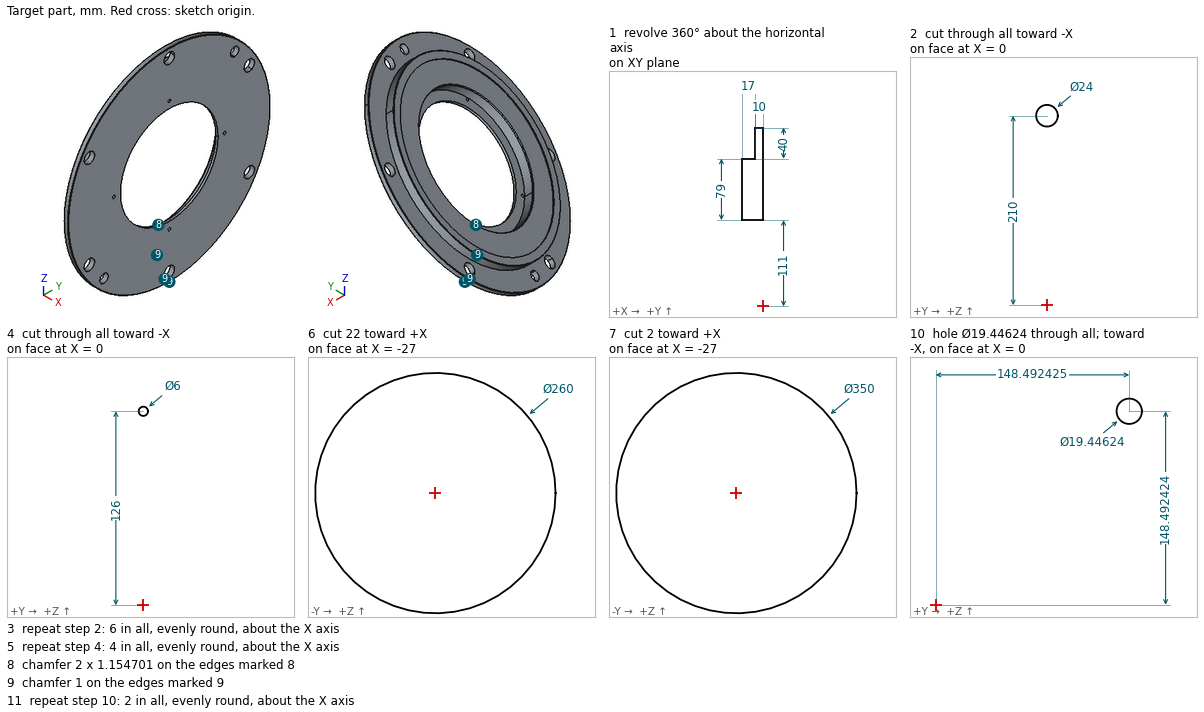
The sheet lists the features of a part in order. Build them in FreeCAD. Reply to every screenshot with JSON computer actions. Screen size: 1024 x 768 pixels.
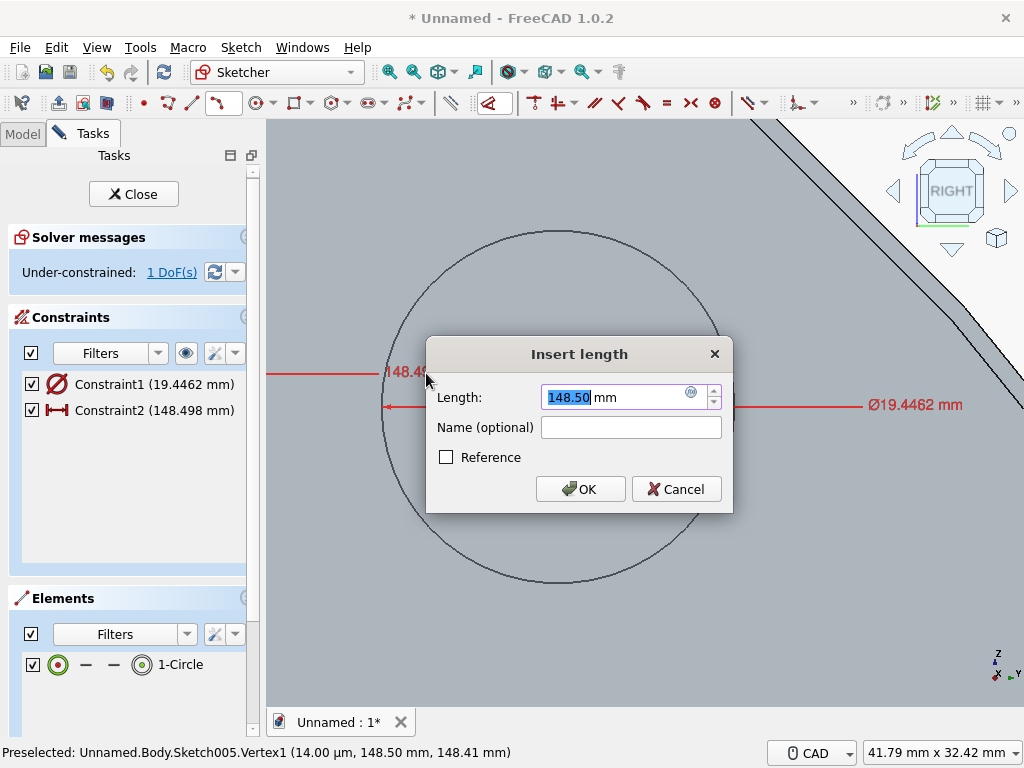
{"action": "type", "text": "148.492425"}
{"action": "key", "text": "Return"}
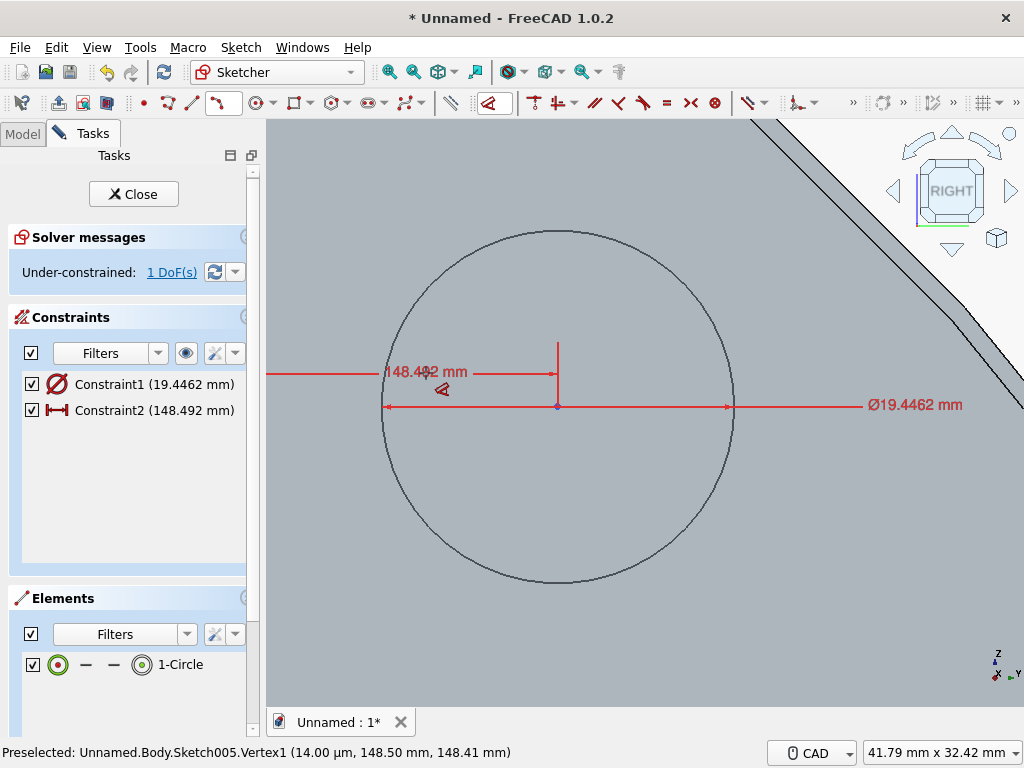
{"action": "left_click", "coordinate": [558, 407]}
{"action": "left_click", "coordinate": [592, 543]}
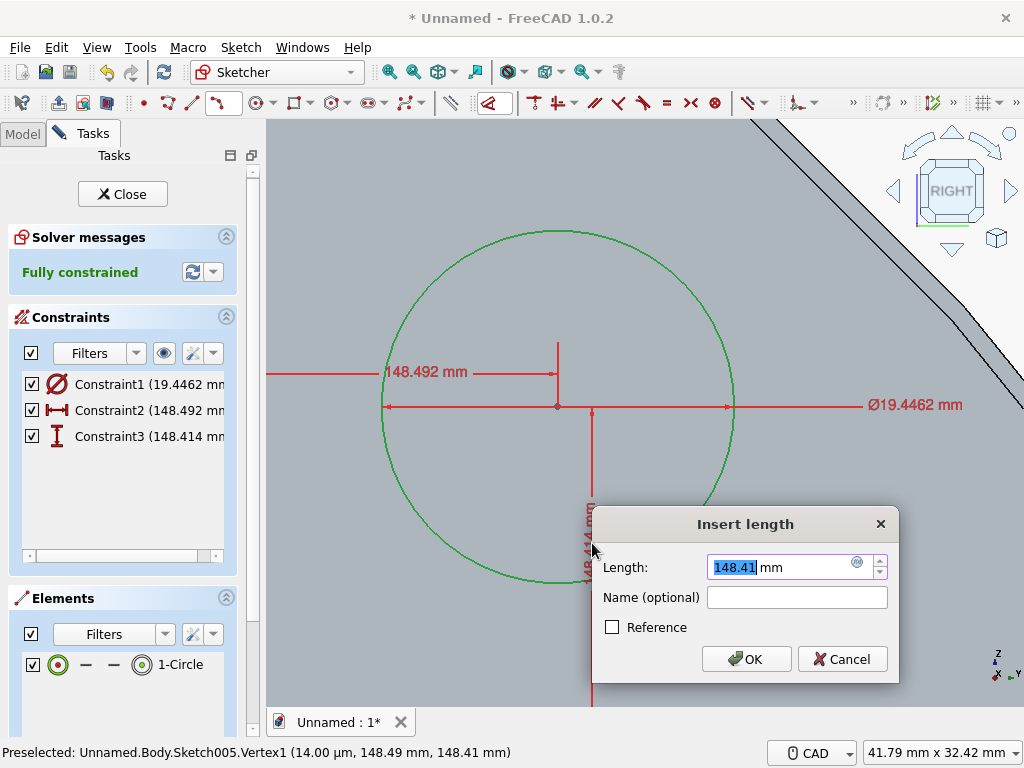
{"action": "type", "text": "148.492424"}
{"action": "key", "text": "Return"}
{"action": "key", "text": "Escape"}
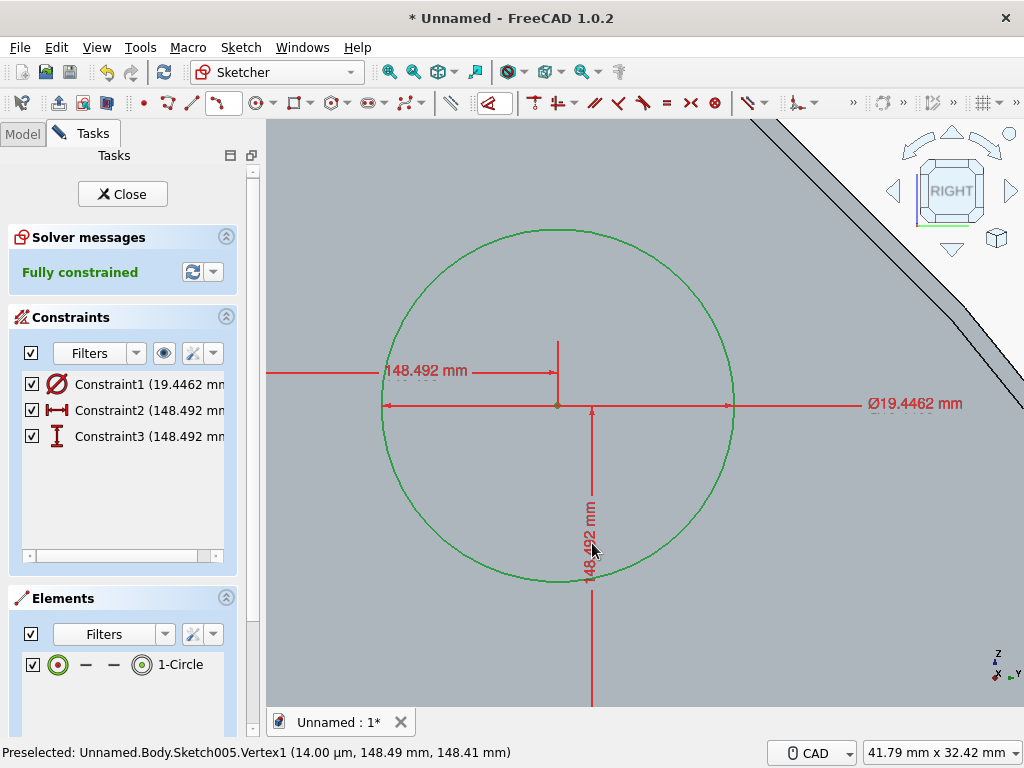
{"action": "left_click", "coordinate": [123, 194]}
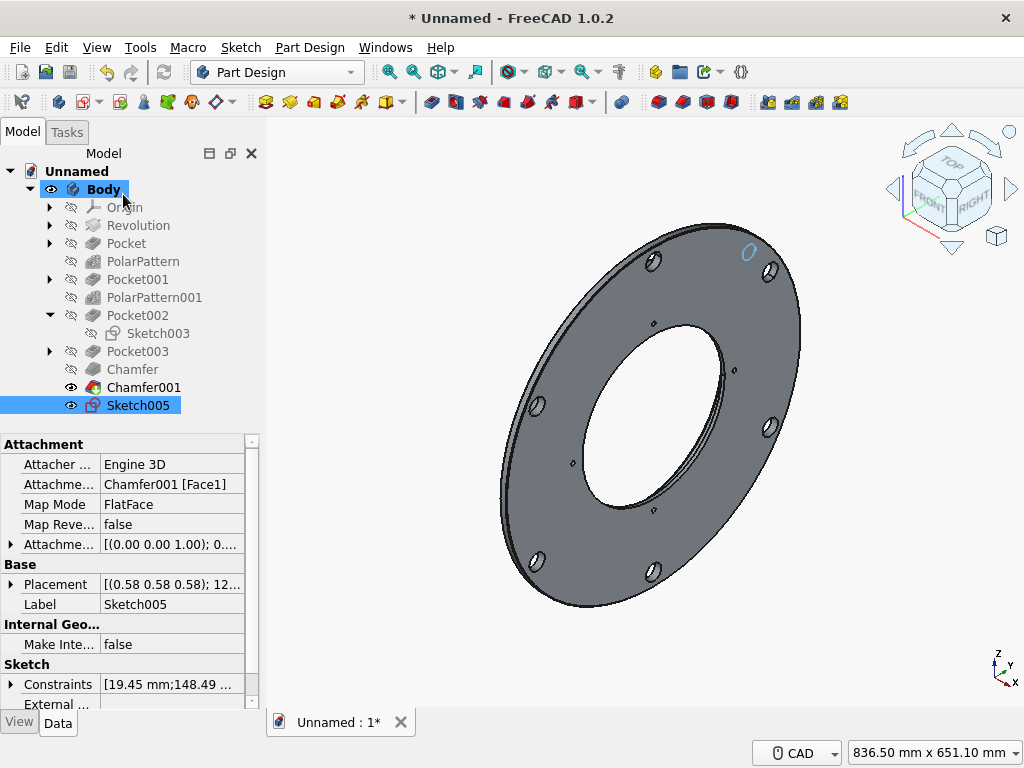
{"action": "left_click", "coordinate": [456, 102]}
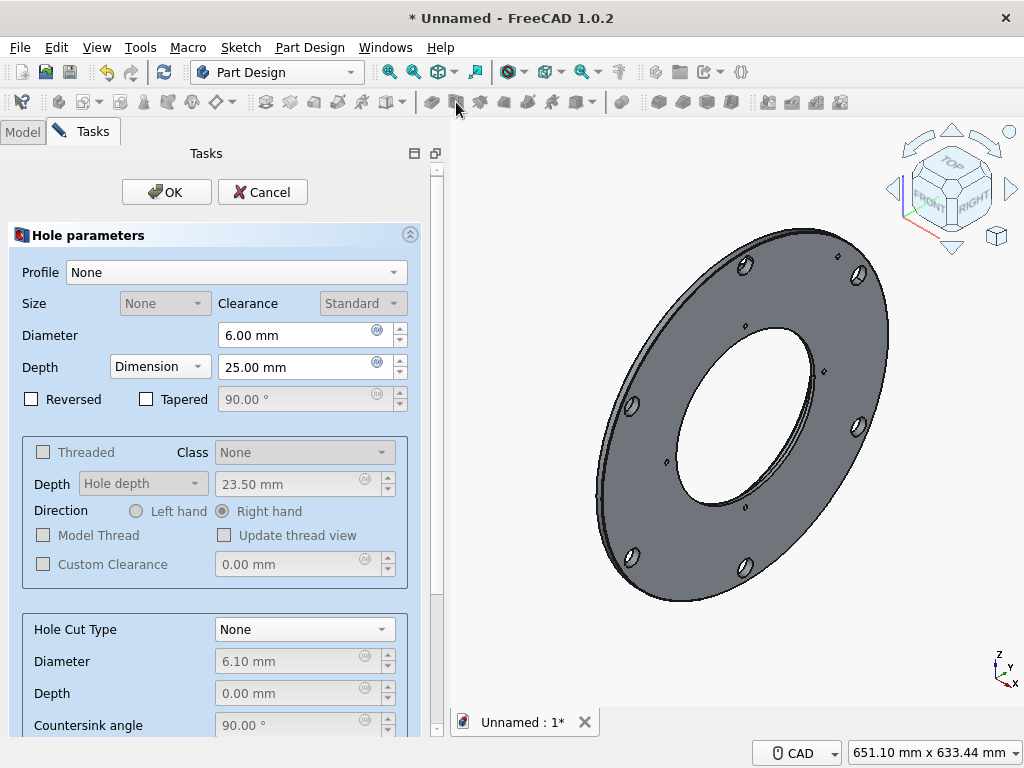
{"action": "triple_click", "coordinate": [305, 335]}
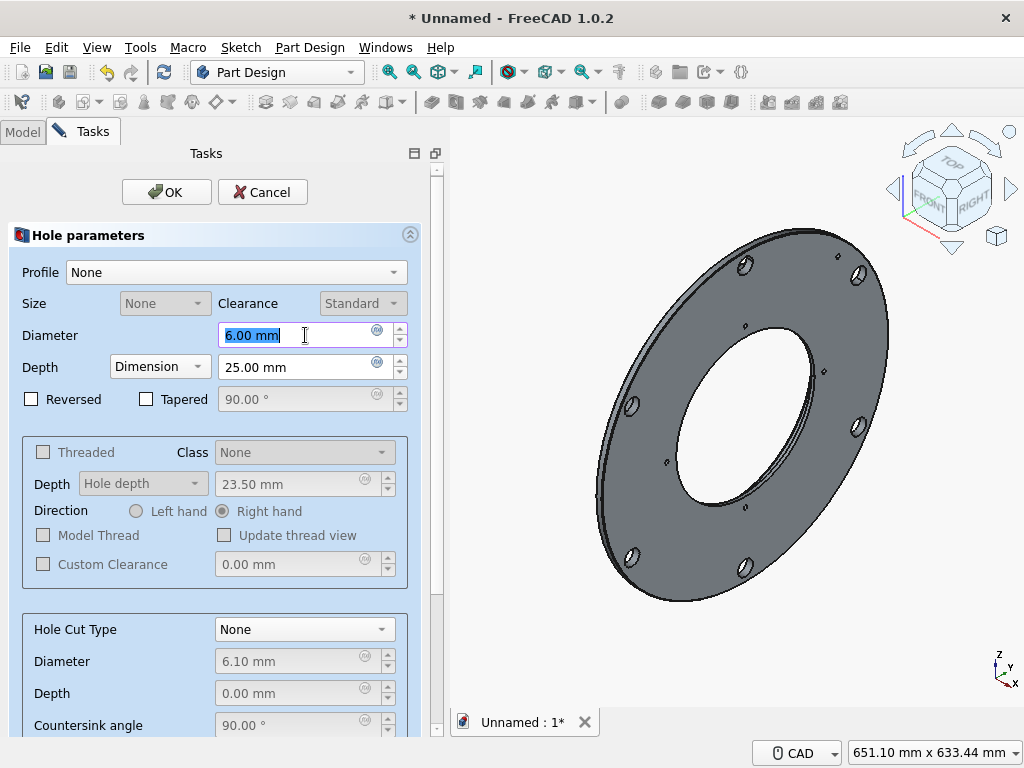
{"action": "type", "text": "19.44624"}
{"action": "key", "text": "Tab"}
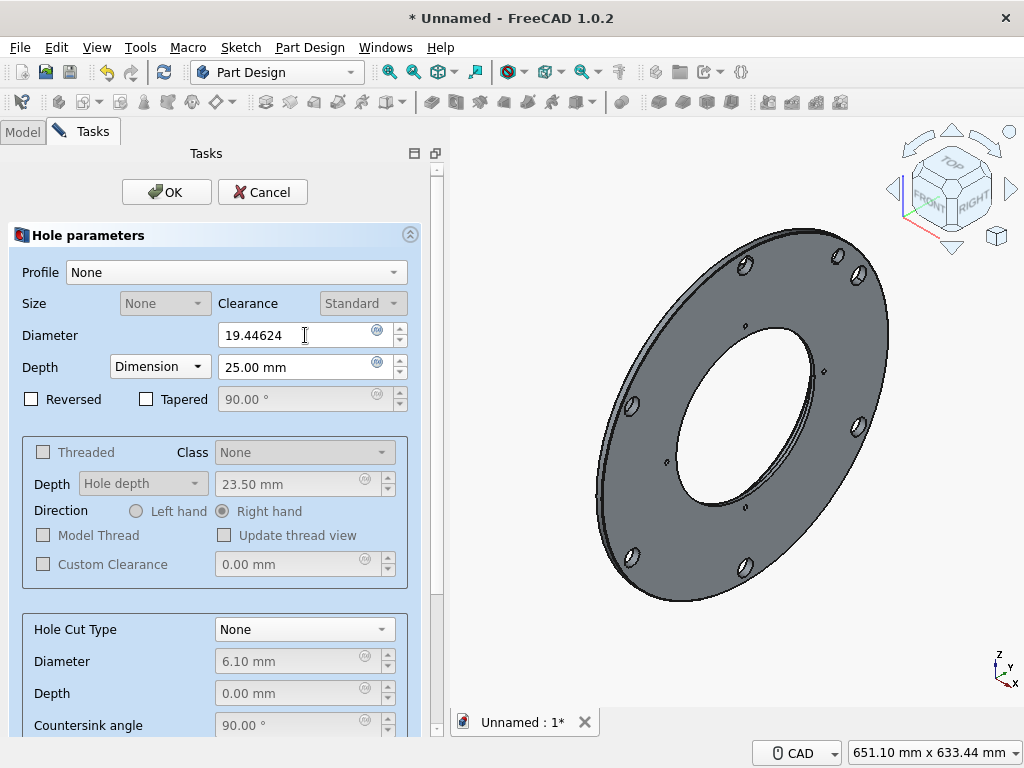
{"action": "left_click", "coordinate": [161, 366]}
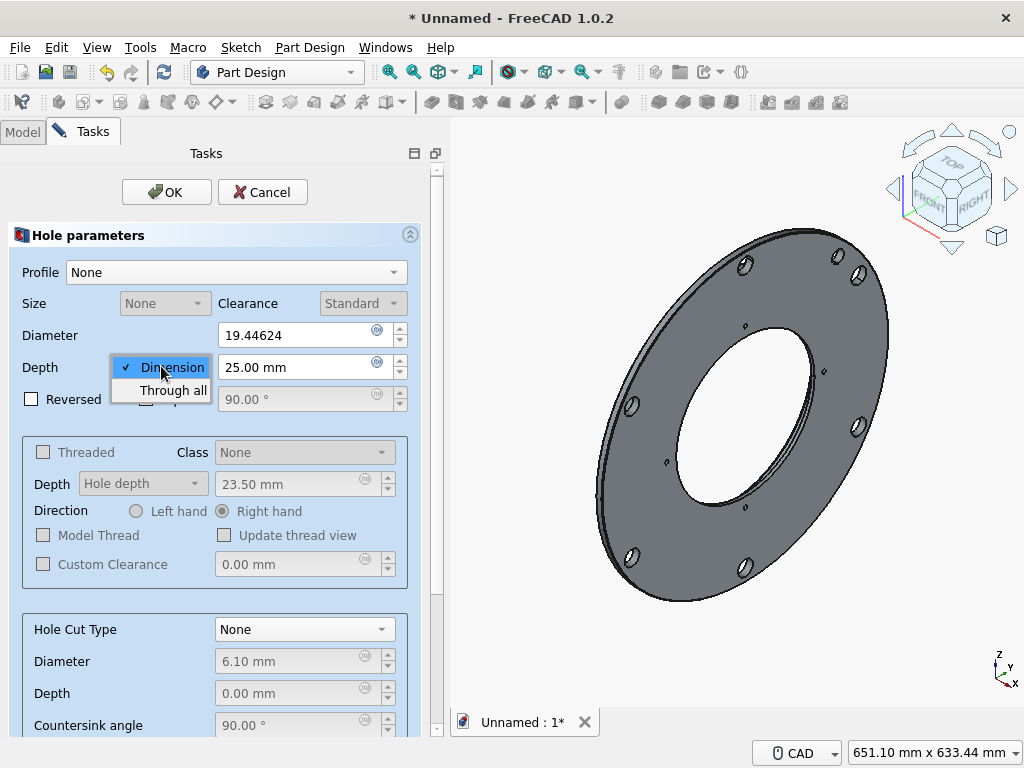
{"action": "left_click", "coordinate": [160, 390]}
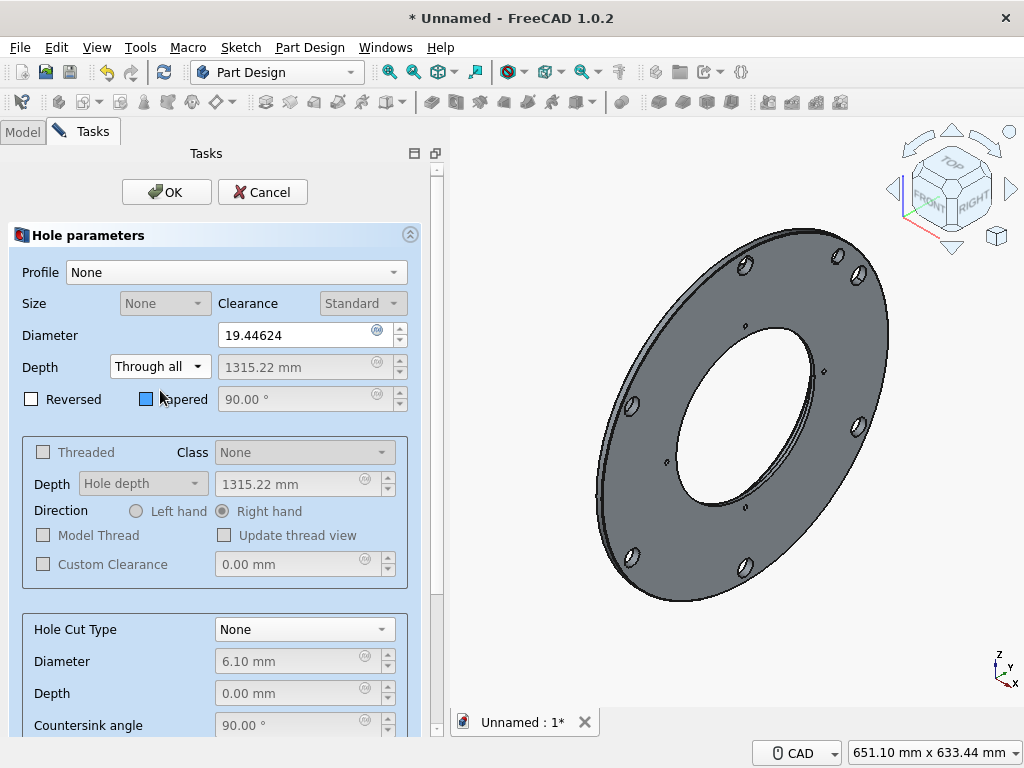
{"action": "left_click", "coordinate": [167, 192]}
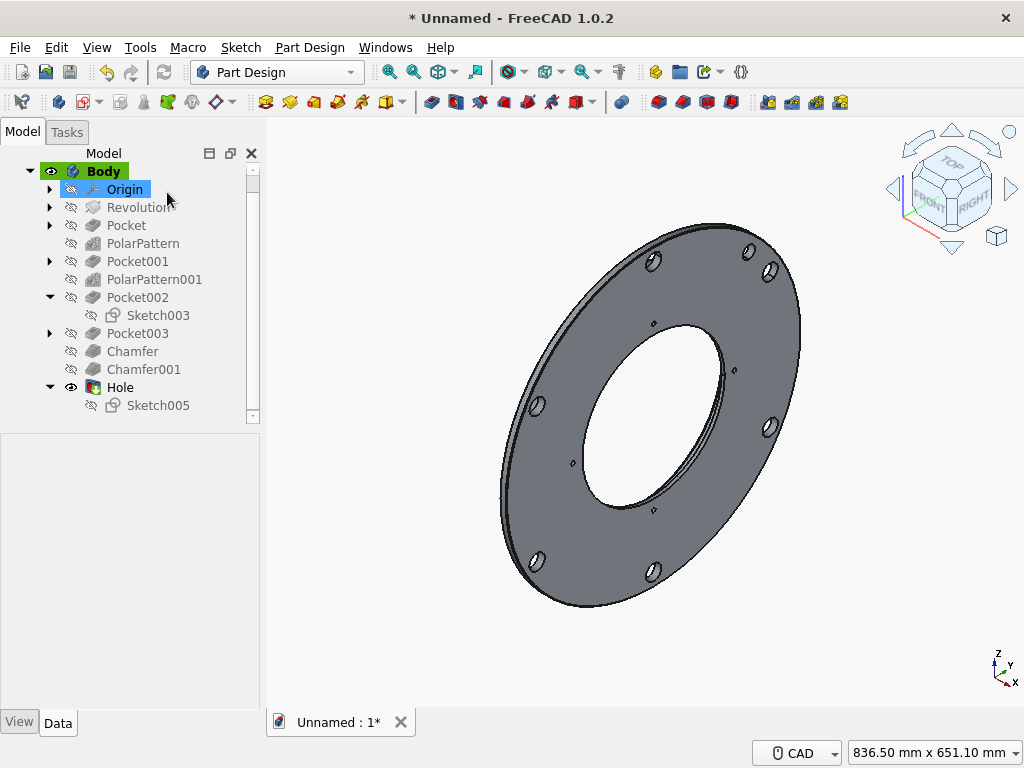
{"action": "left_click", "coordinate": [116, 387]}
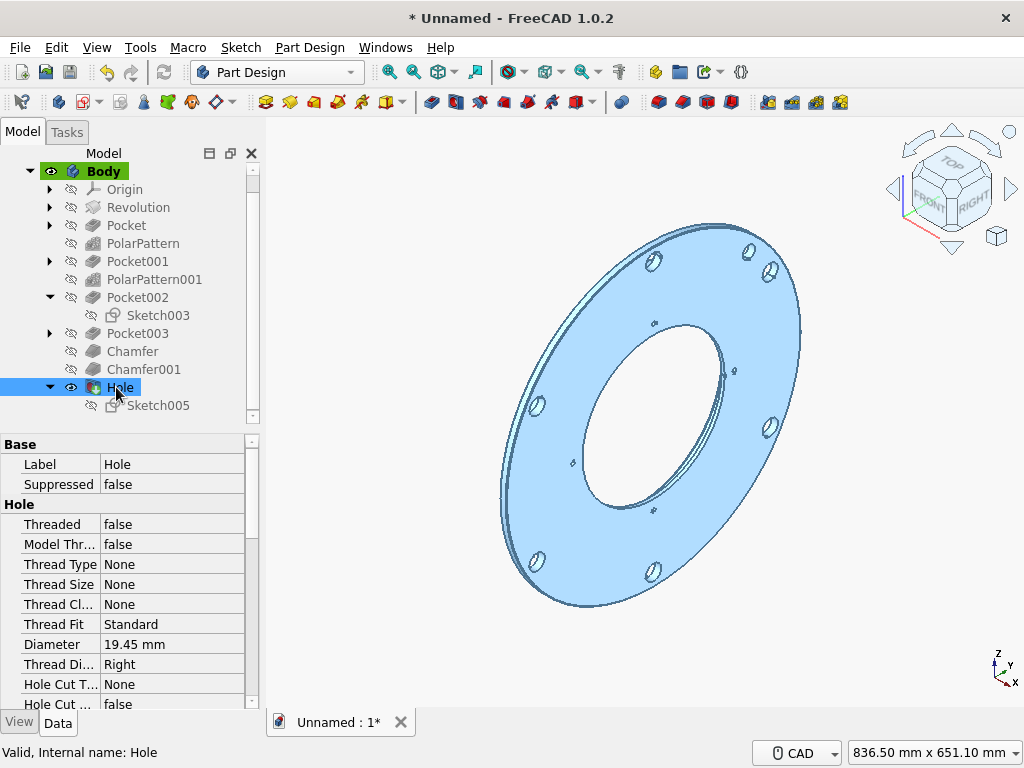
{"action": "left_click", "coordinate": [816, 102]}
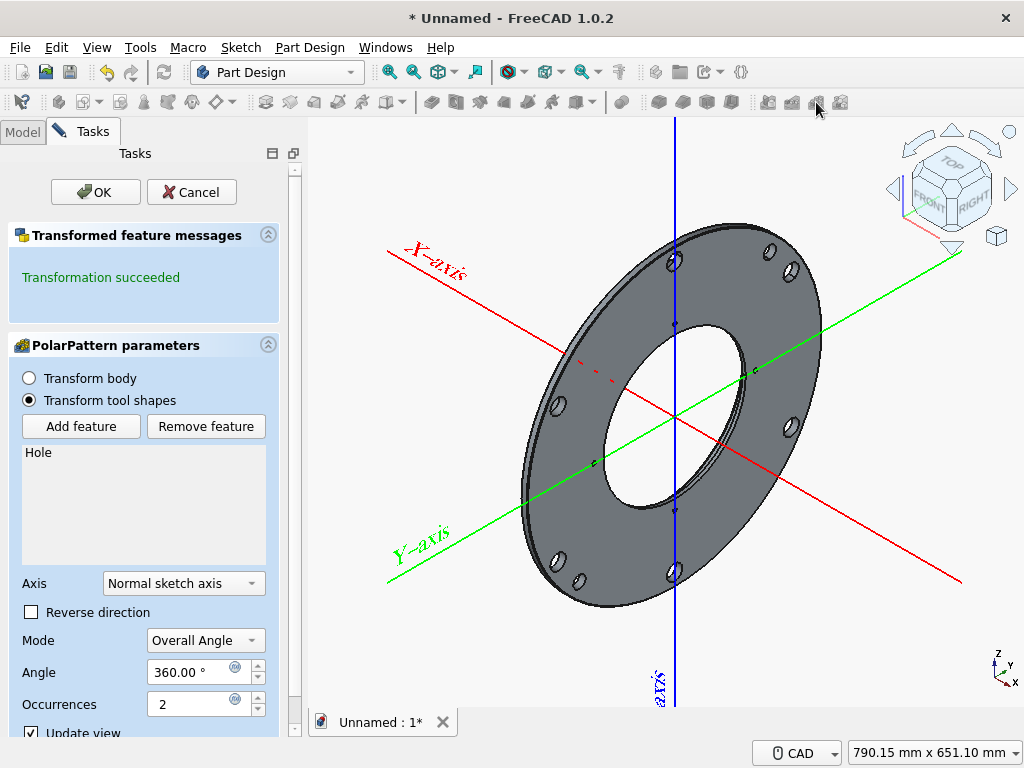
{"action": "left_click", "coordinate": [184, 584]}